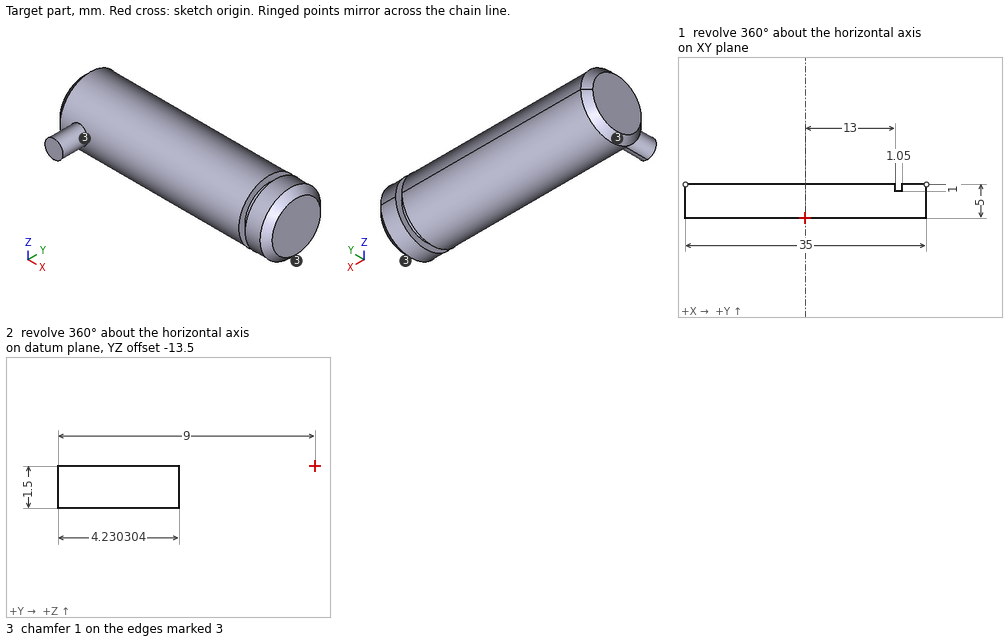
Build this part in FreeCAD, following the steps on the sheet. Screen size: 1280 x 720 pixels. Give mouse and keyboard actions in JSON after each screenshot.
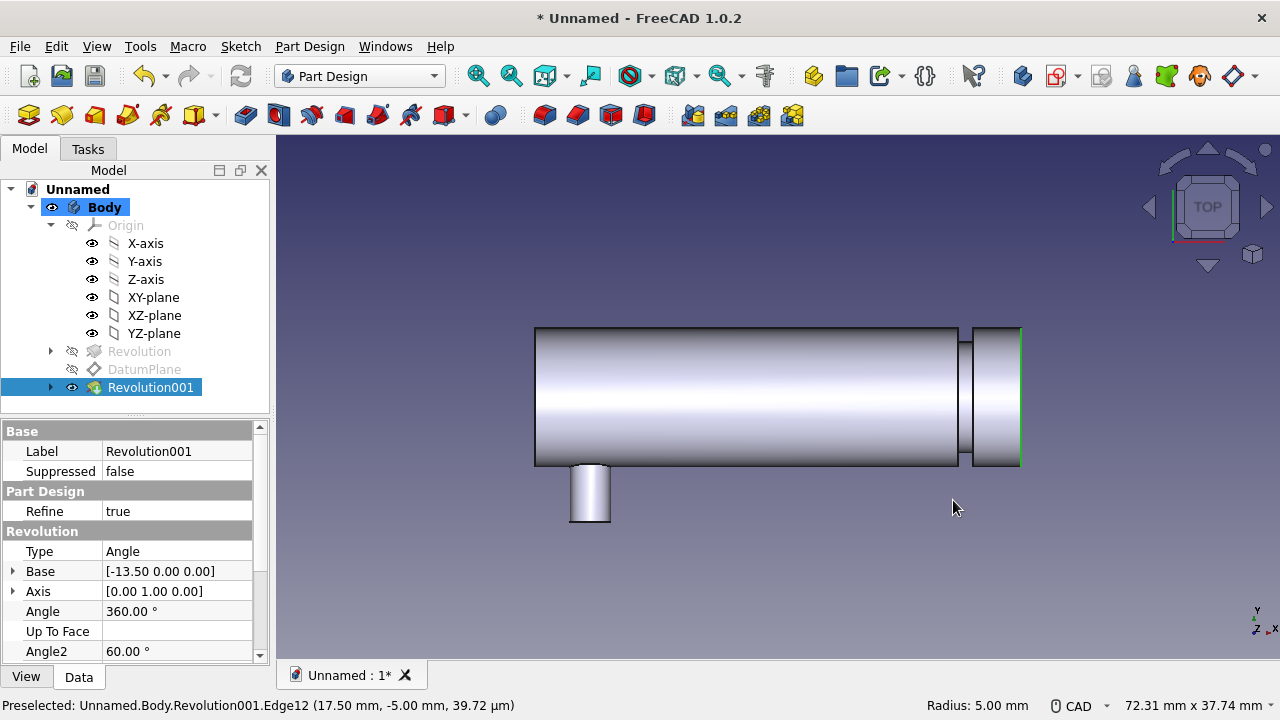
{"action": "left_click", "coordinate": [535, 418], "text": "ctrl"}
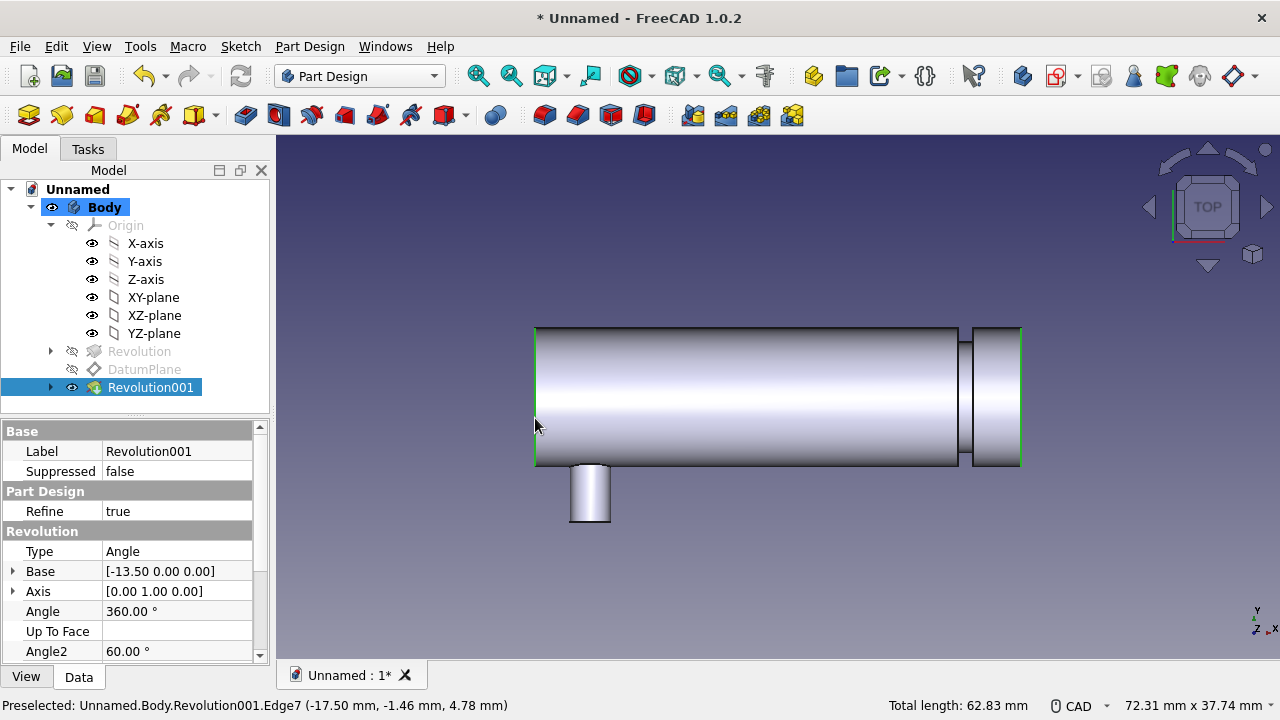
{"action": "left_click", "coordinate": [578, 116]}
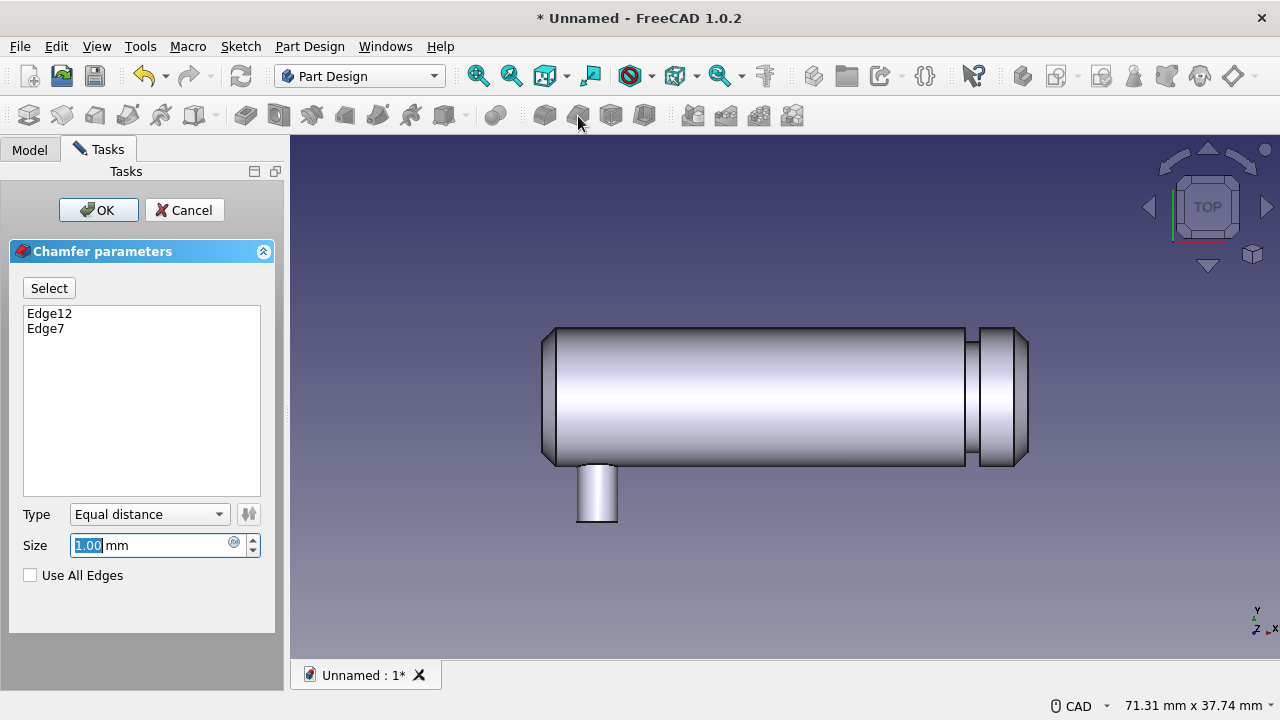
{"action": "type", "text": "1"}
{"action": "key", "text": "Tab"}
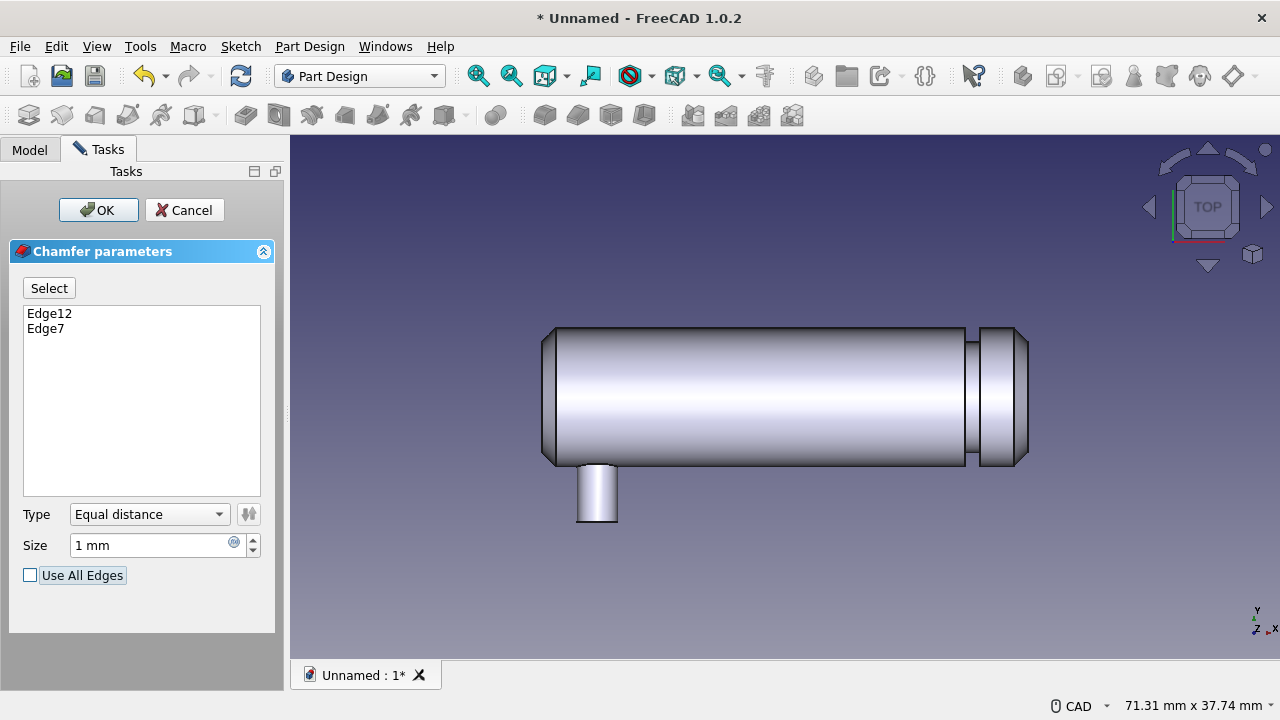
{"action": "left_click", "coordinate": [99, 210]}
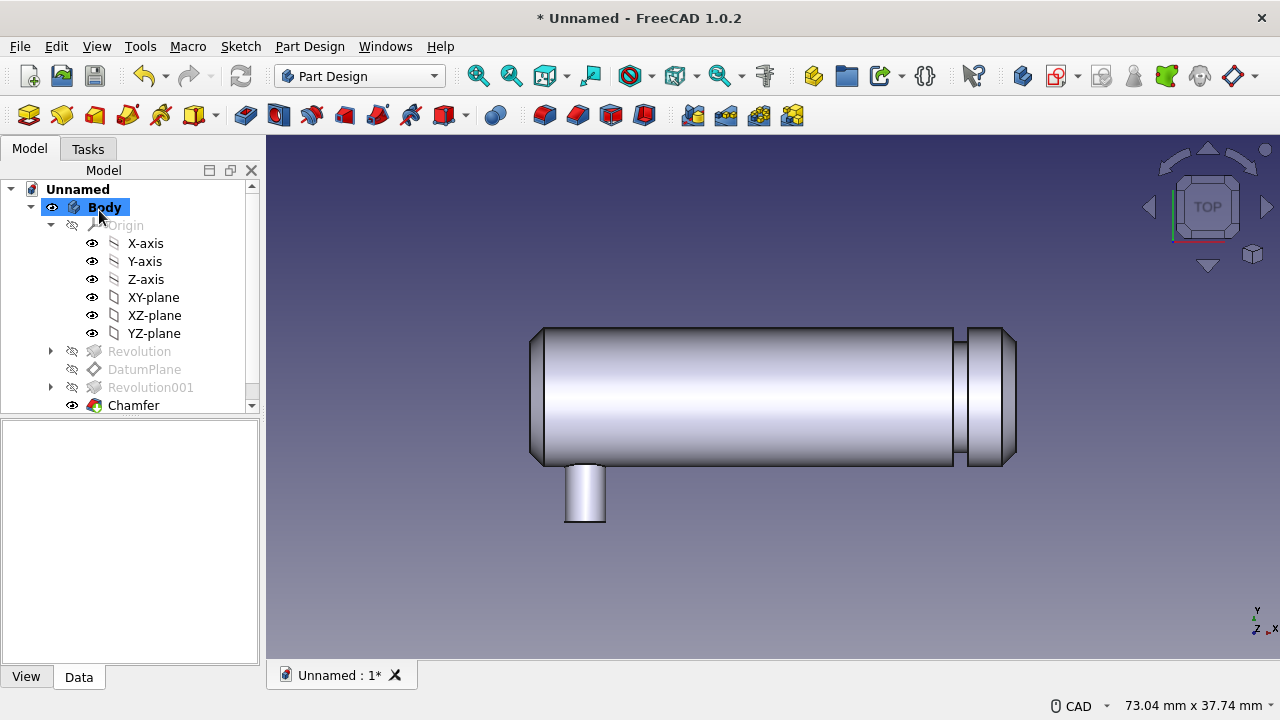
{"action": "key", "text": "0"}